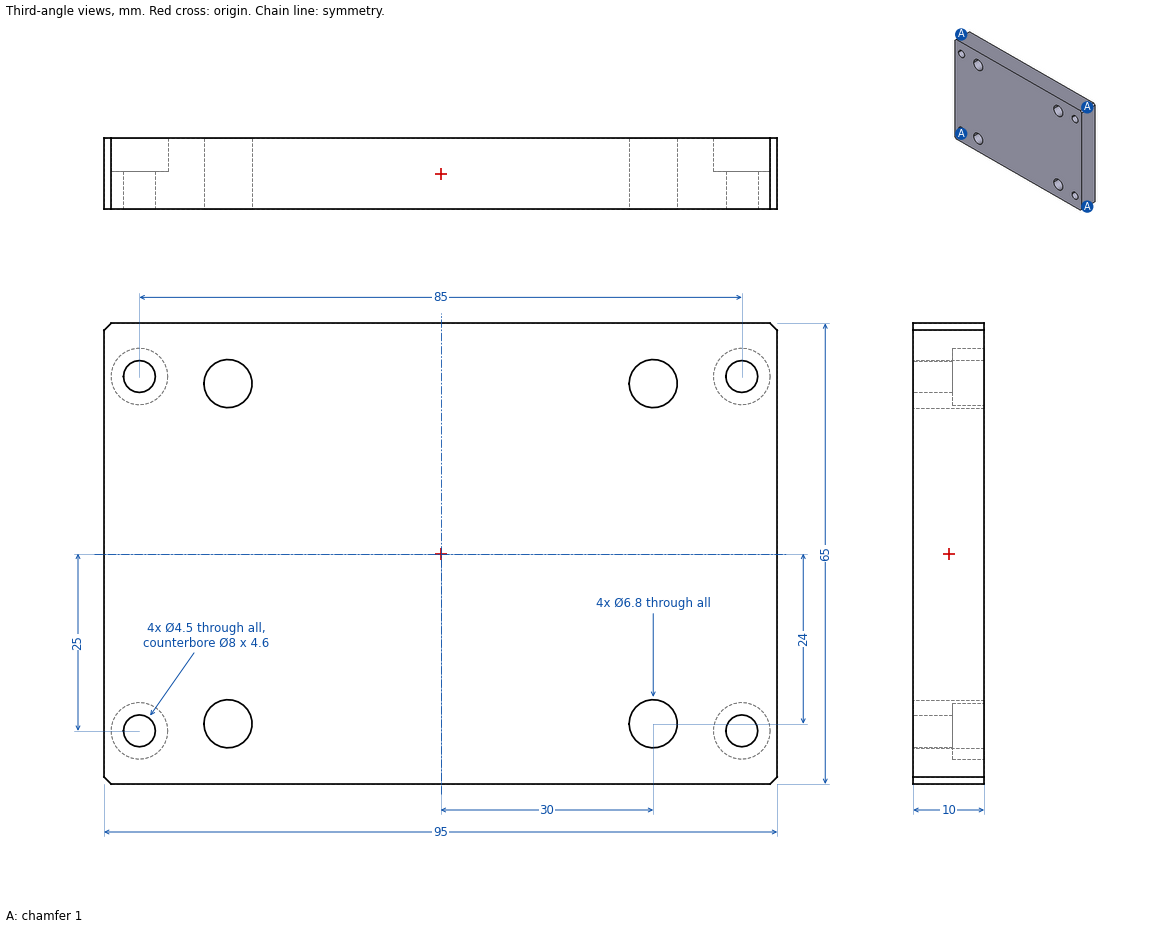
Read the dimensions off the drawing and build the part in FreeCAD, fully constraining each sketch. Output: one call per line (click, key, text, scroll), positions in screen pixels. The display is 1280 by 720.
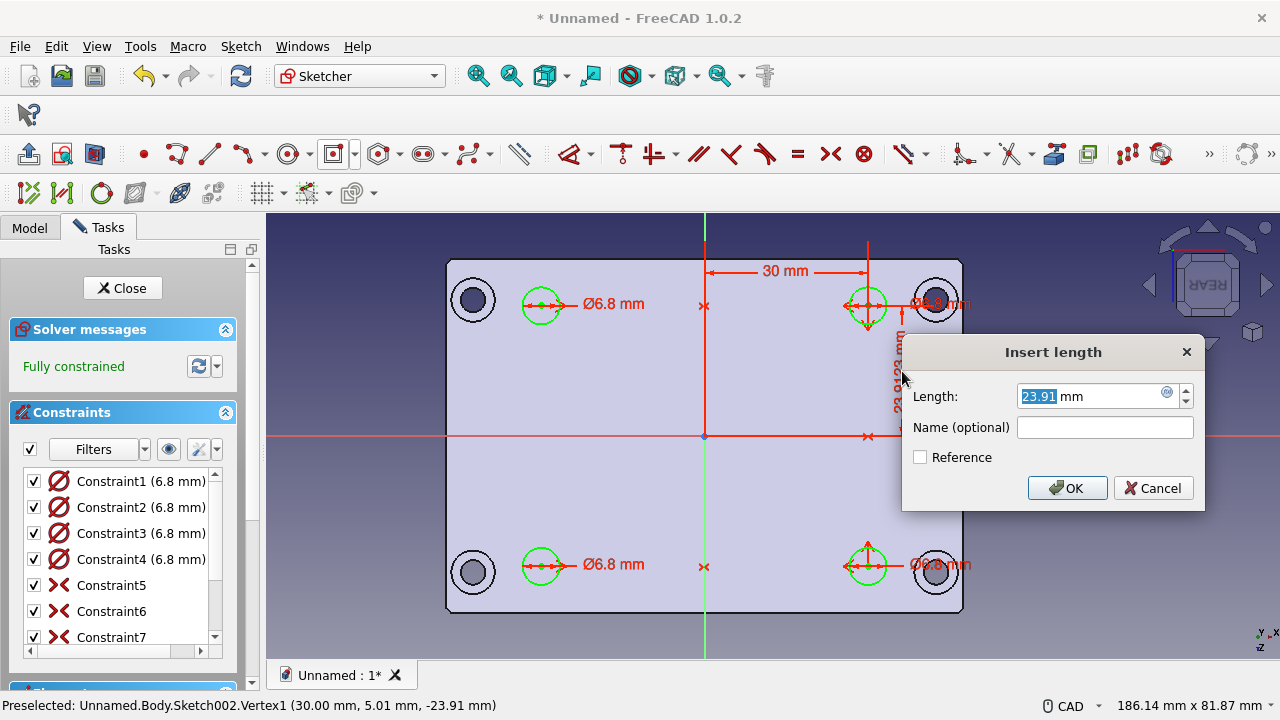
text(24)
key(Return)
key(Escape)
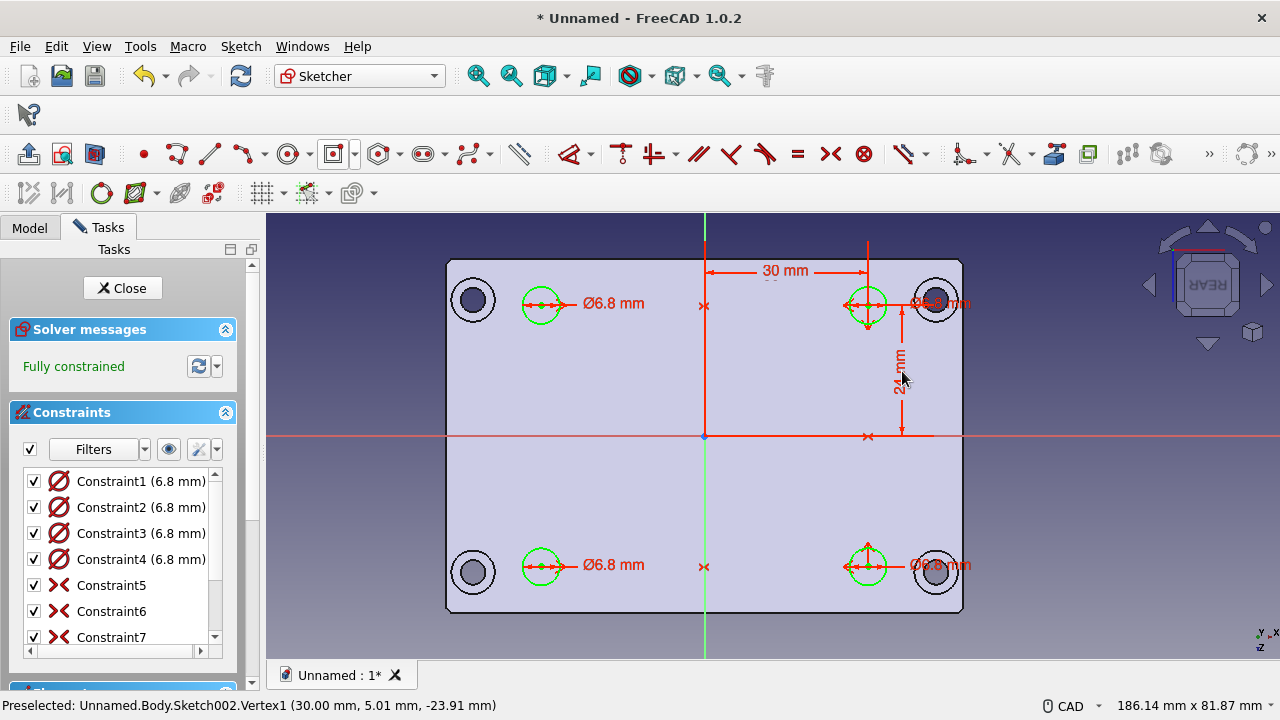
click(123, 288)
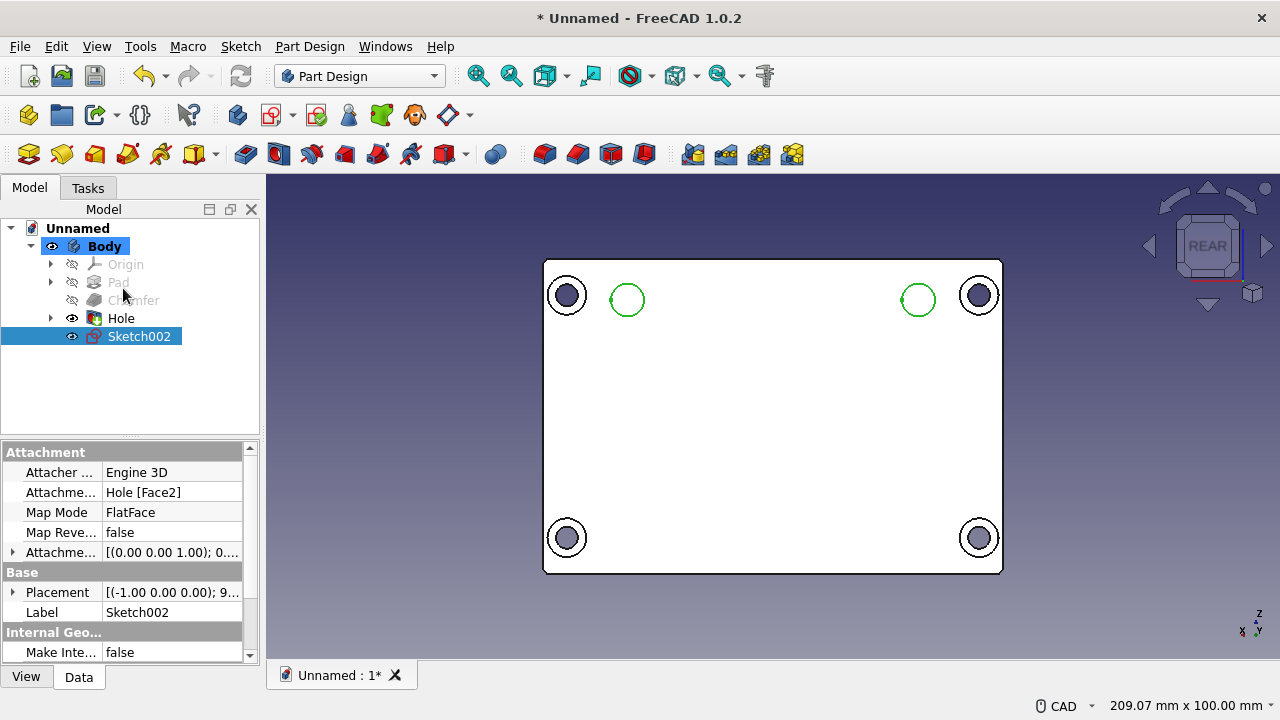
click(279, 154)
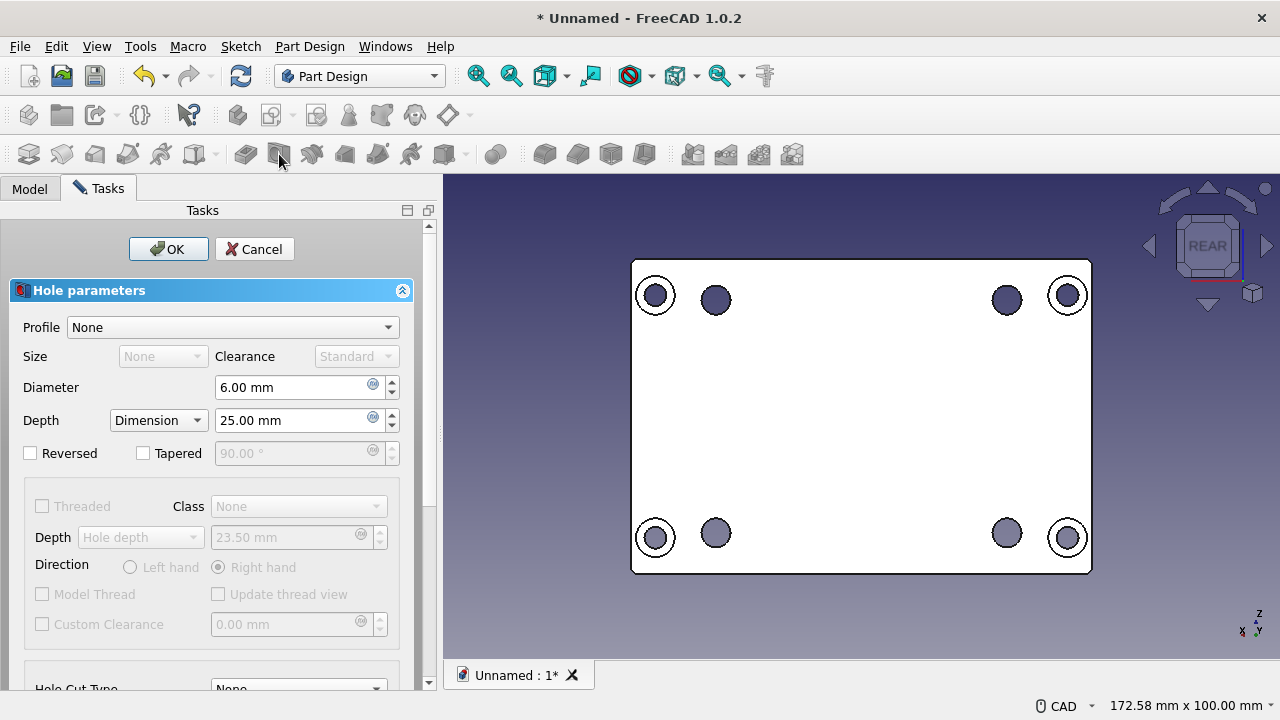
triple_click(300, 388)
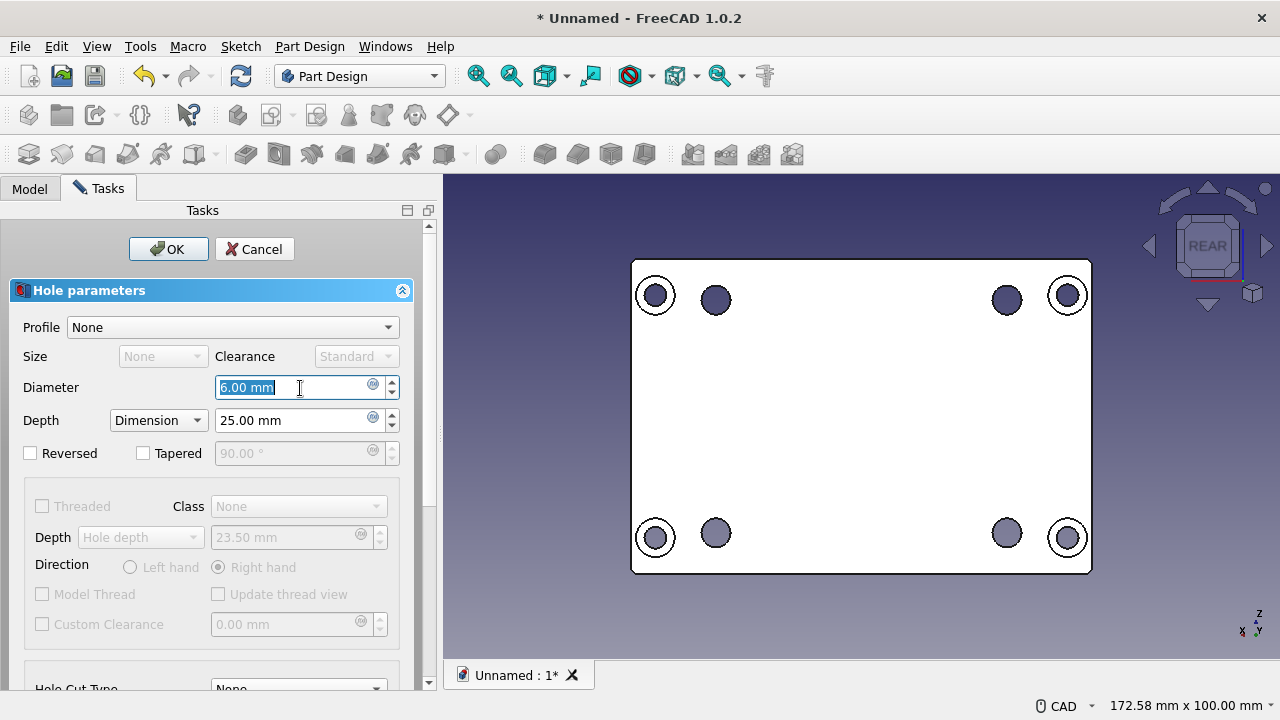
text(6.8)
key(Tab)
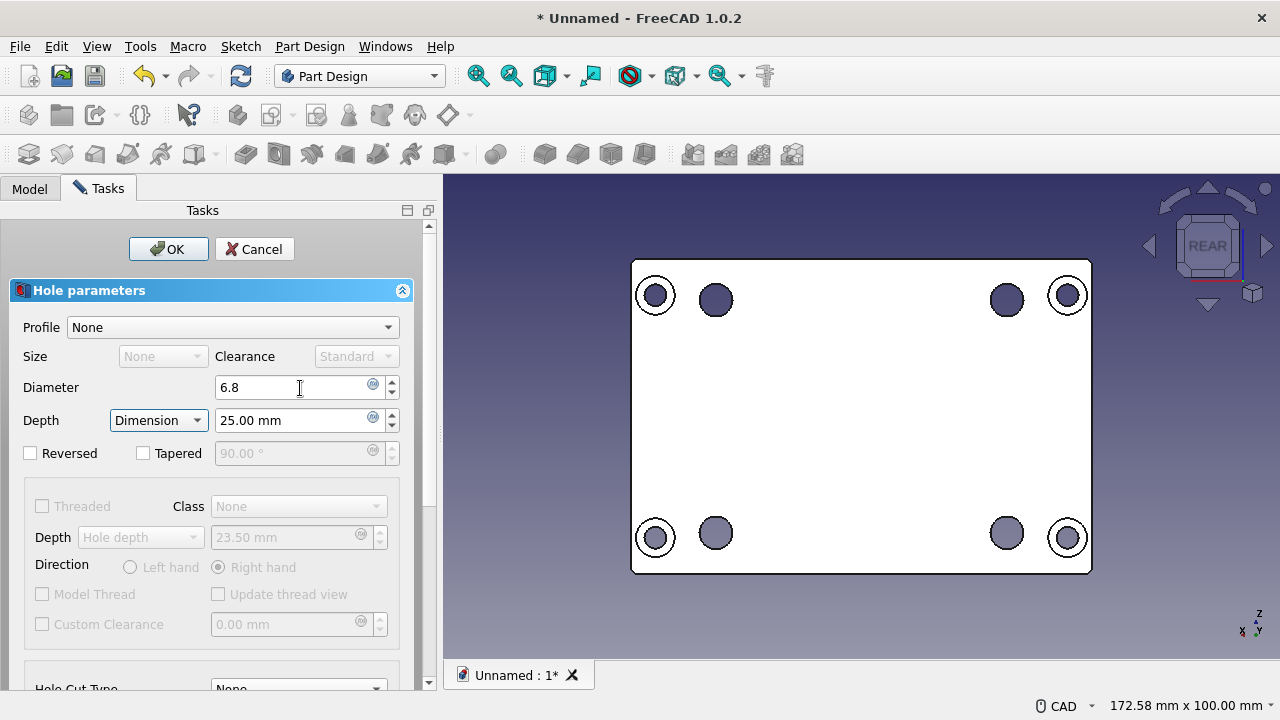
click(160, 420)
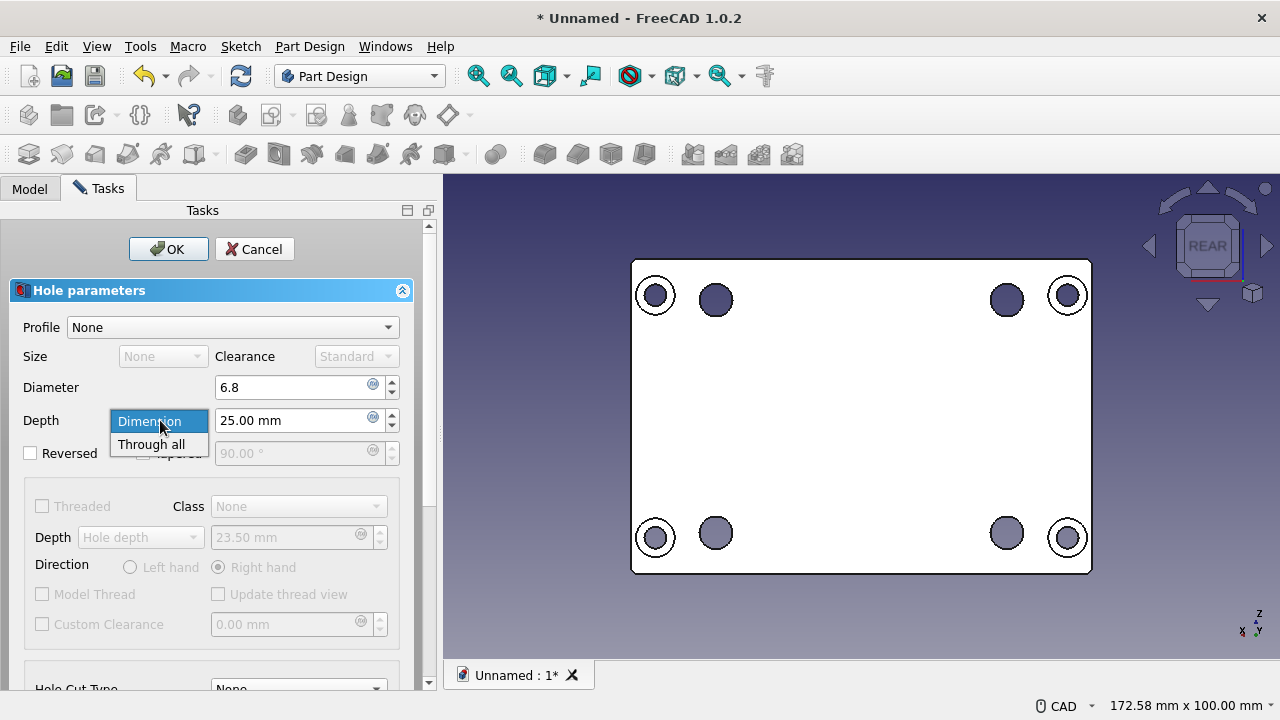
click(158, 444)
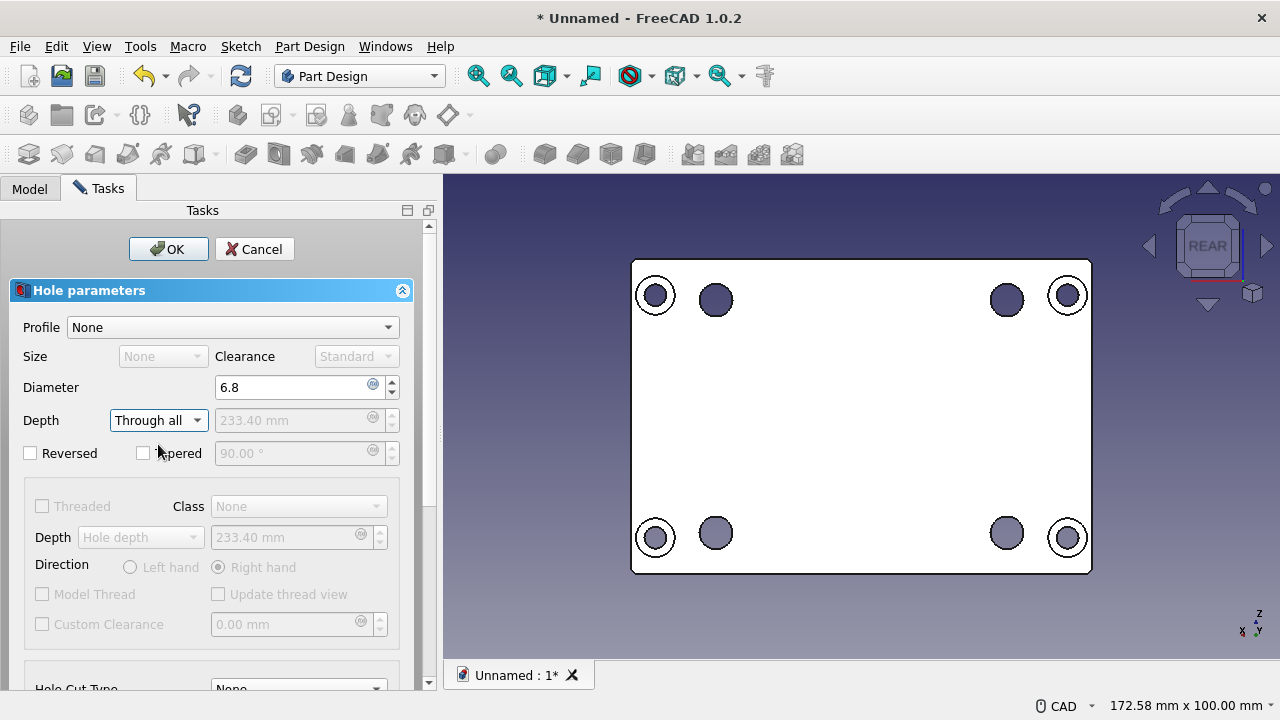
click(169, 249)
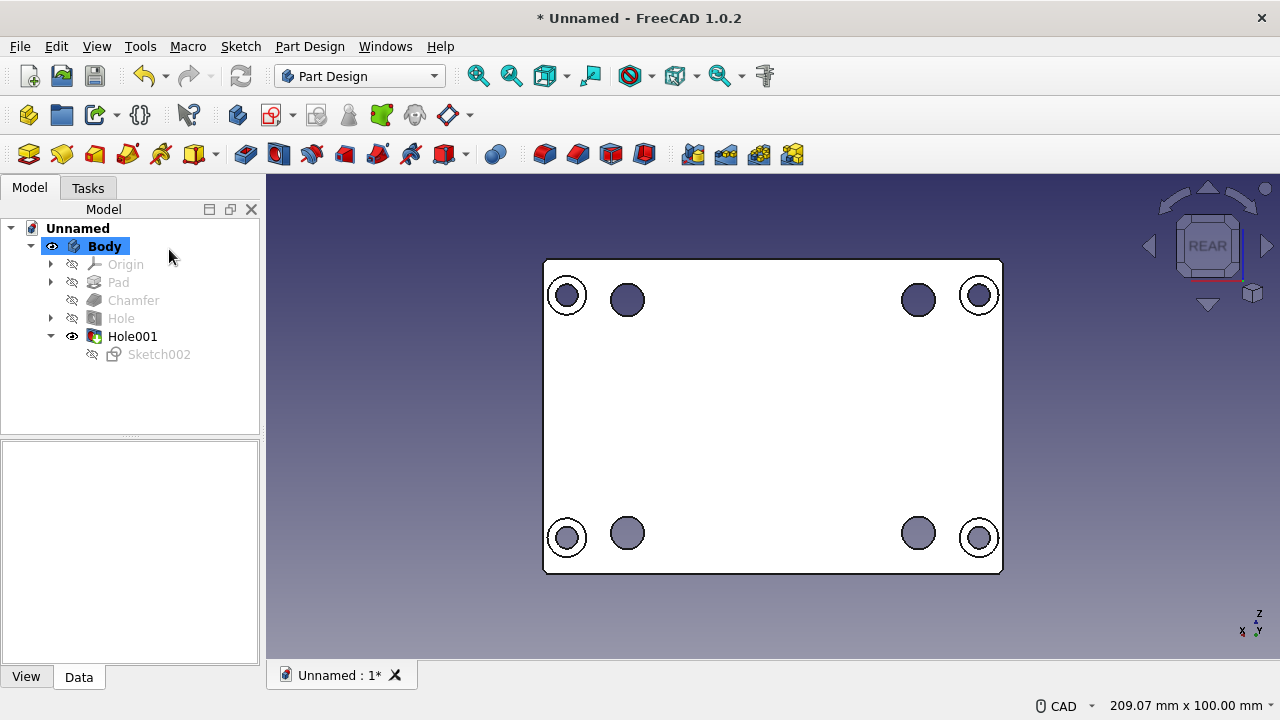
key(0)